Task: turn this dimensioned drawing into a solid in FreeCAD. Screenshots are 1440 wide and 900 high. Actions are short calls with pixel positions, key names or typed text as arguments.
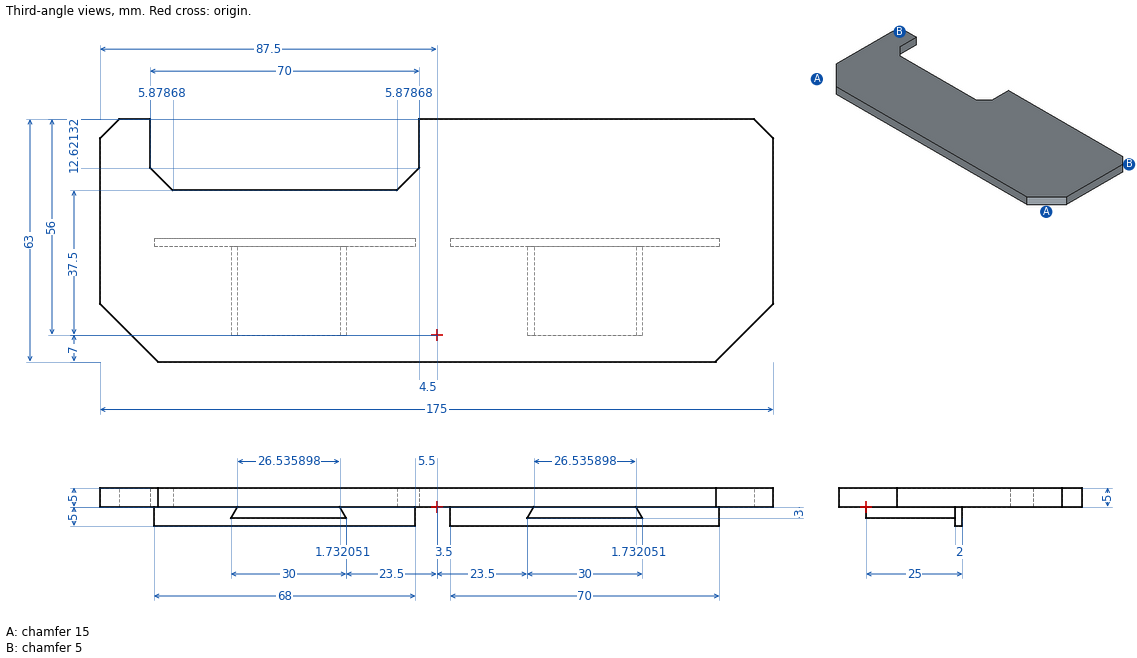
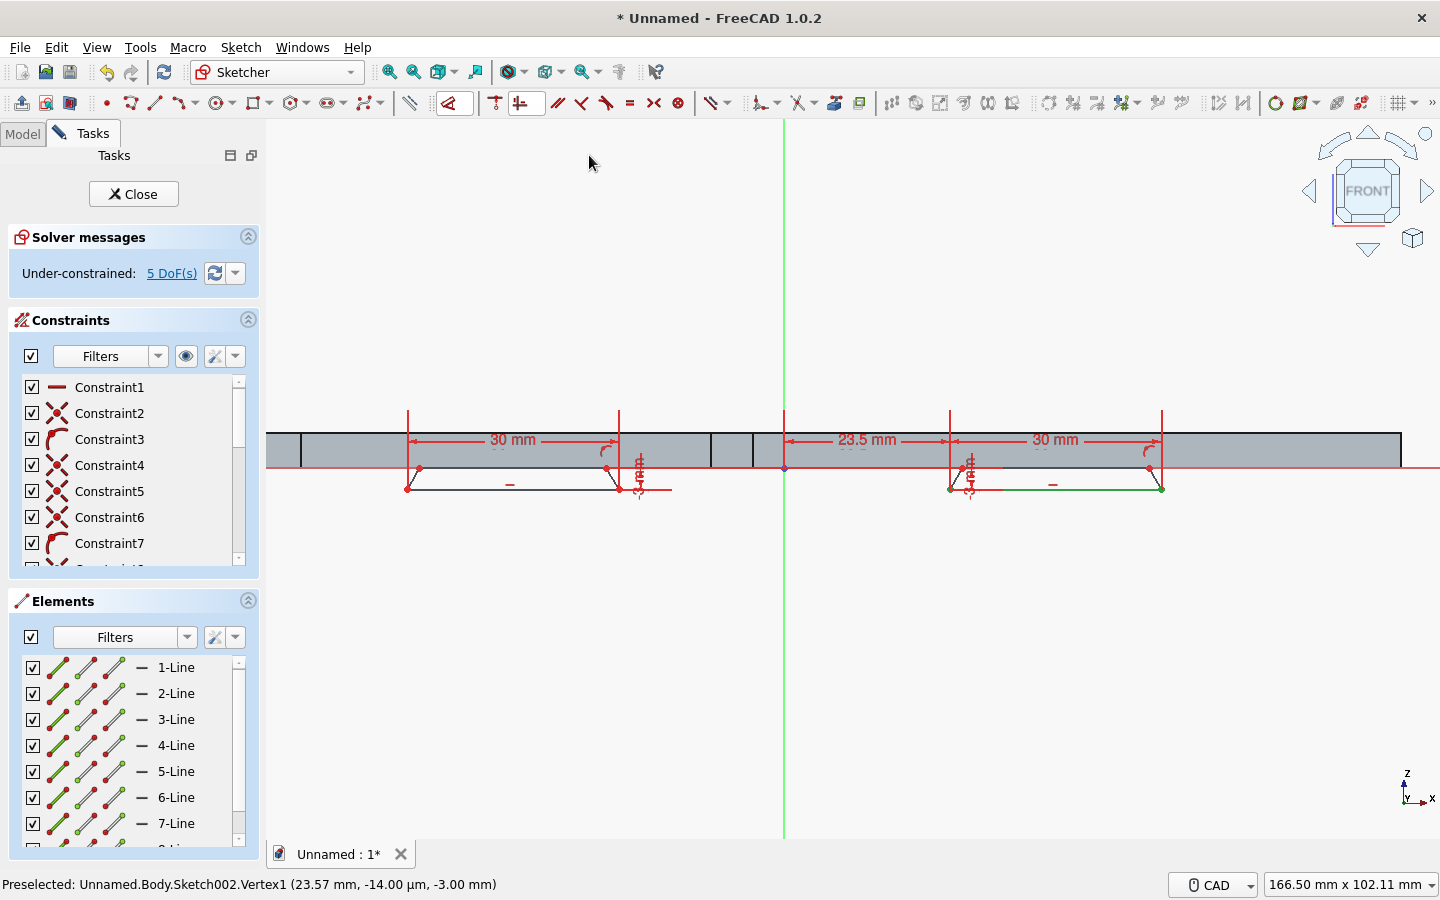
click(619, 490)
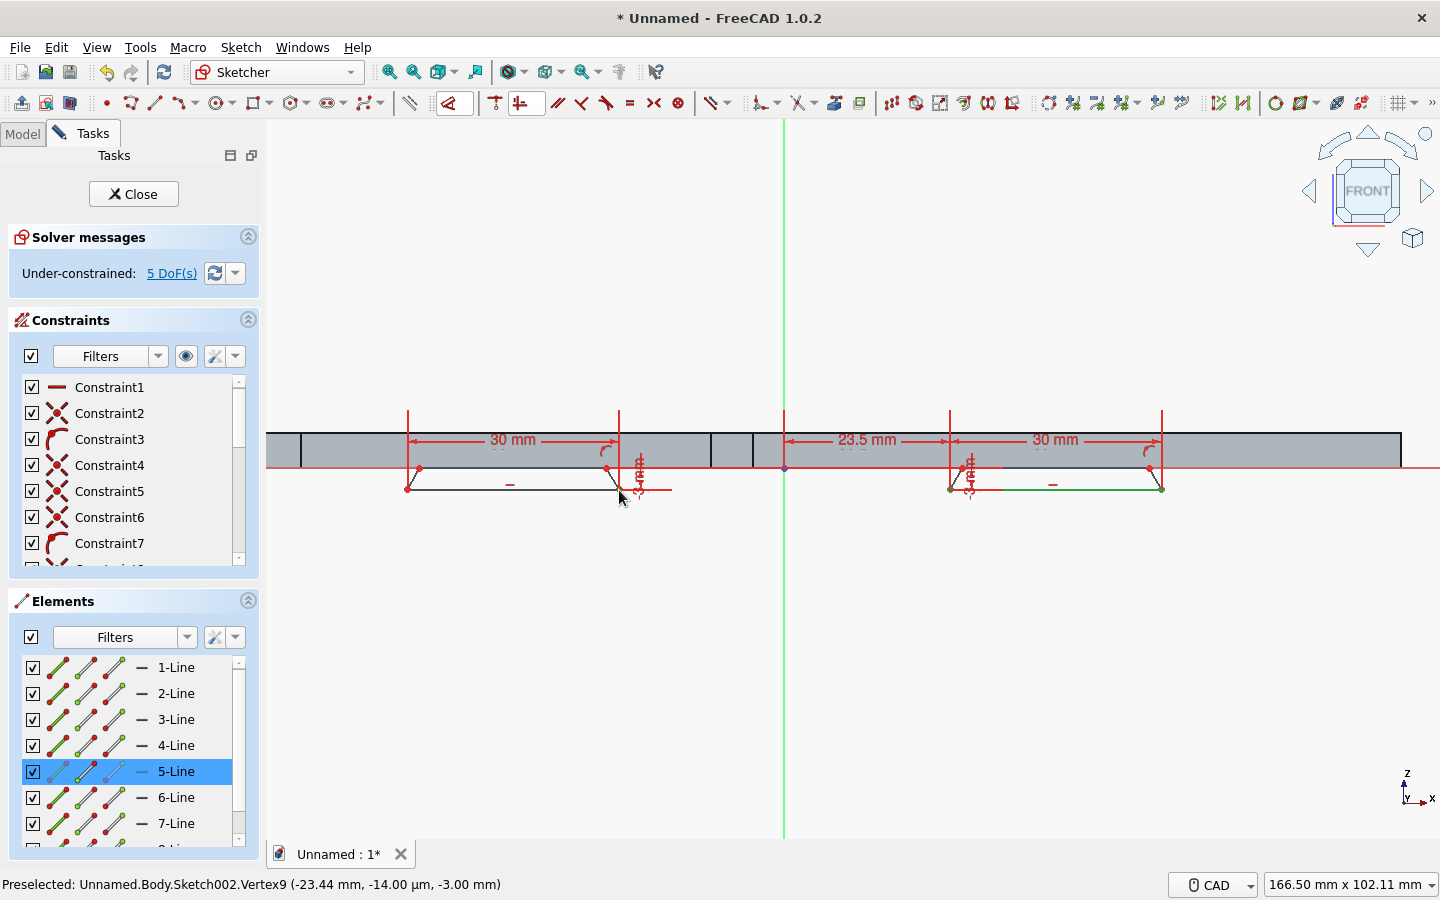
click(468, 104)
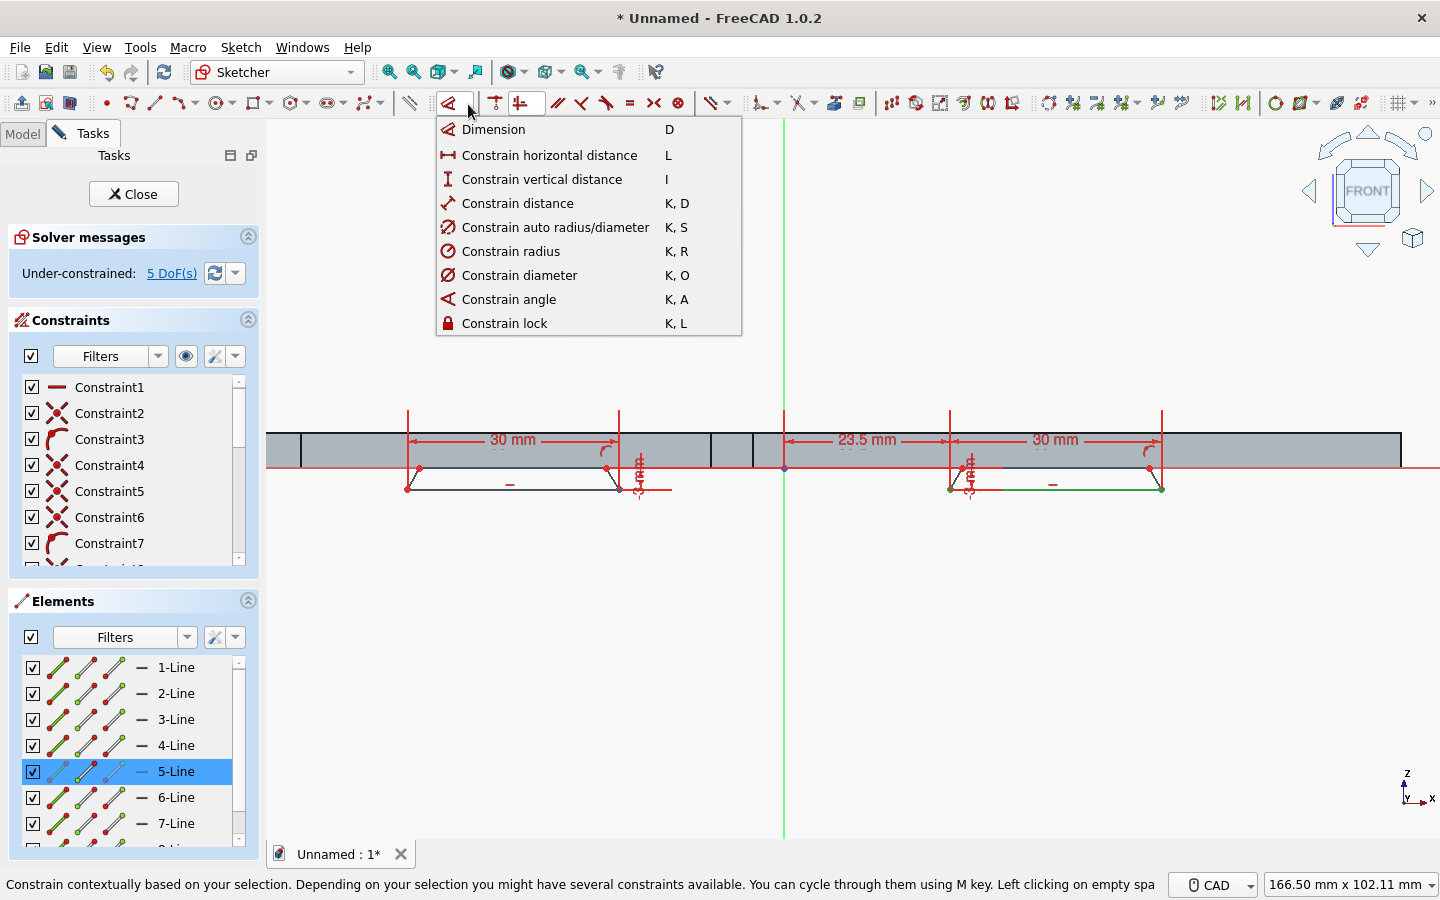
click(589, 155)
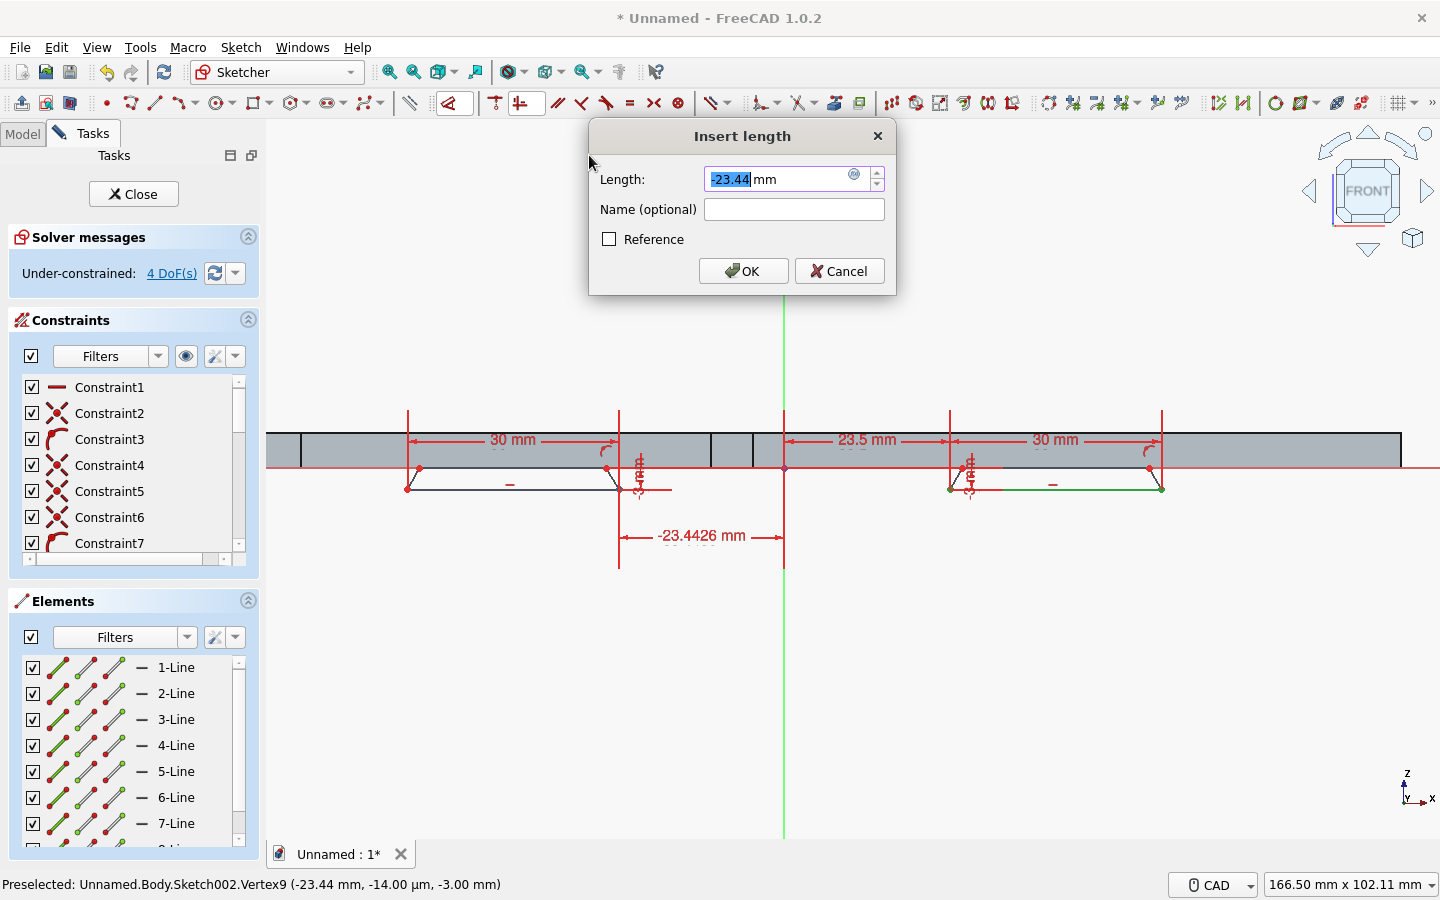
text(-23.5)
key(Return)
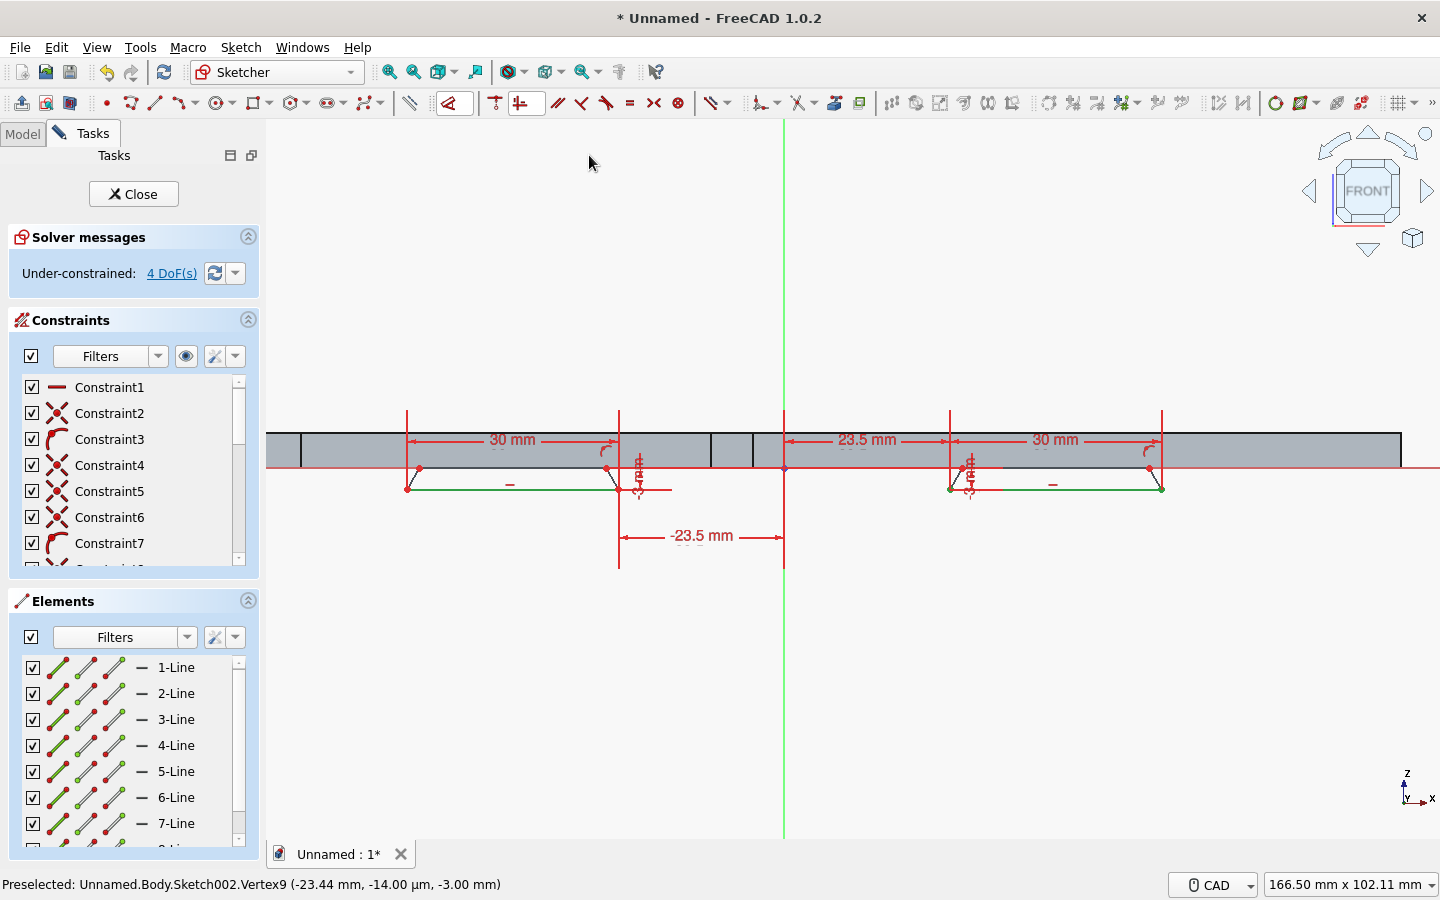
click(1093, 468)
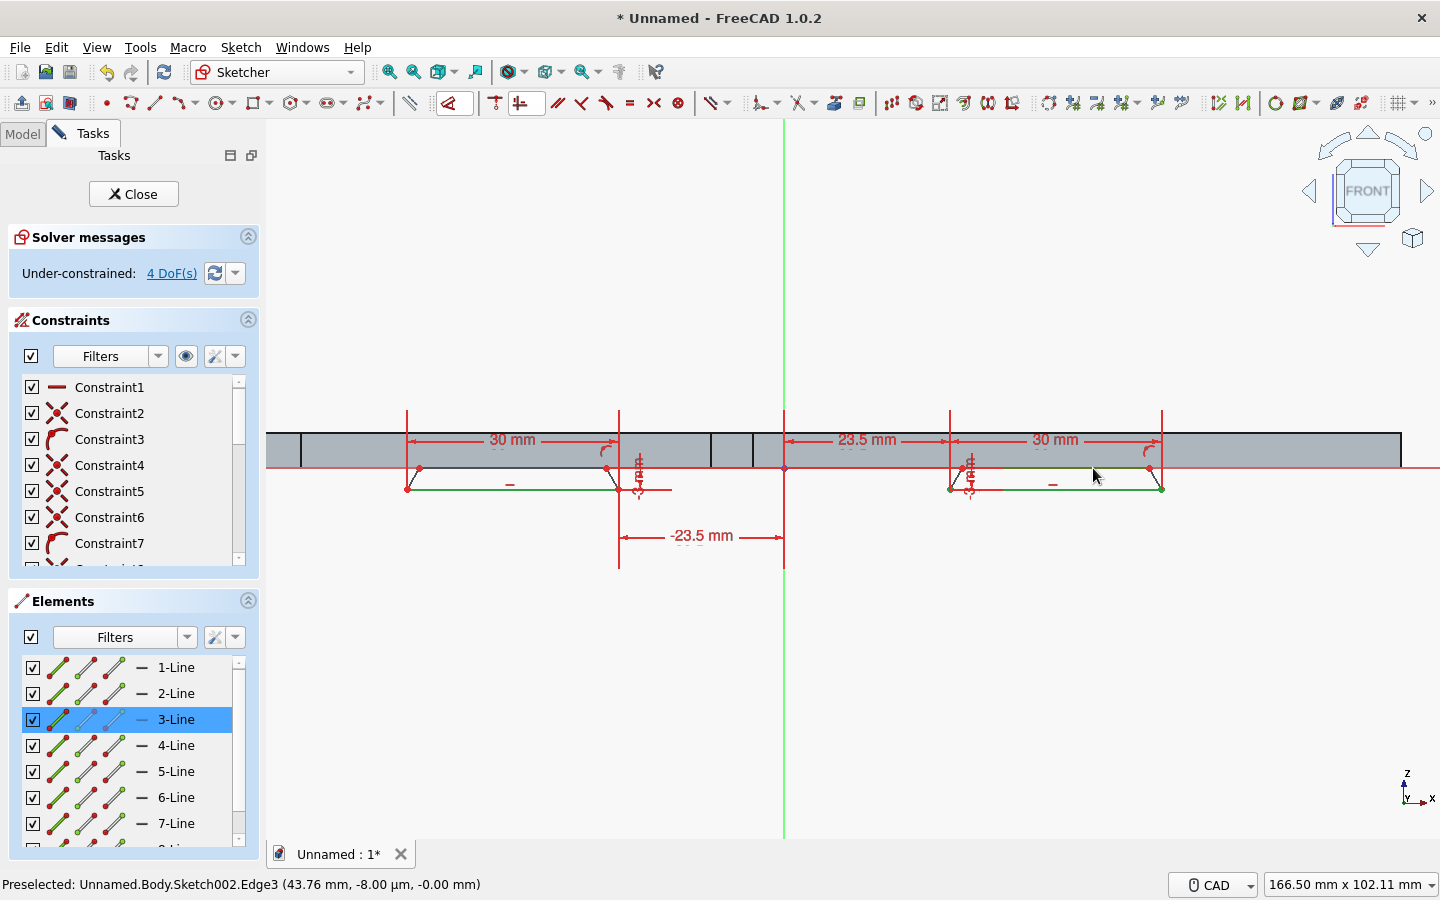
key(l)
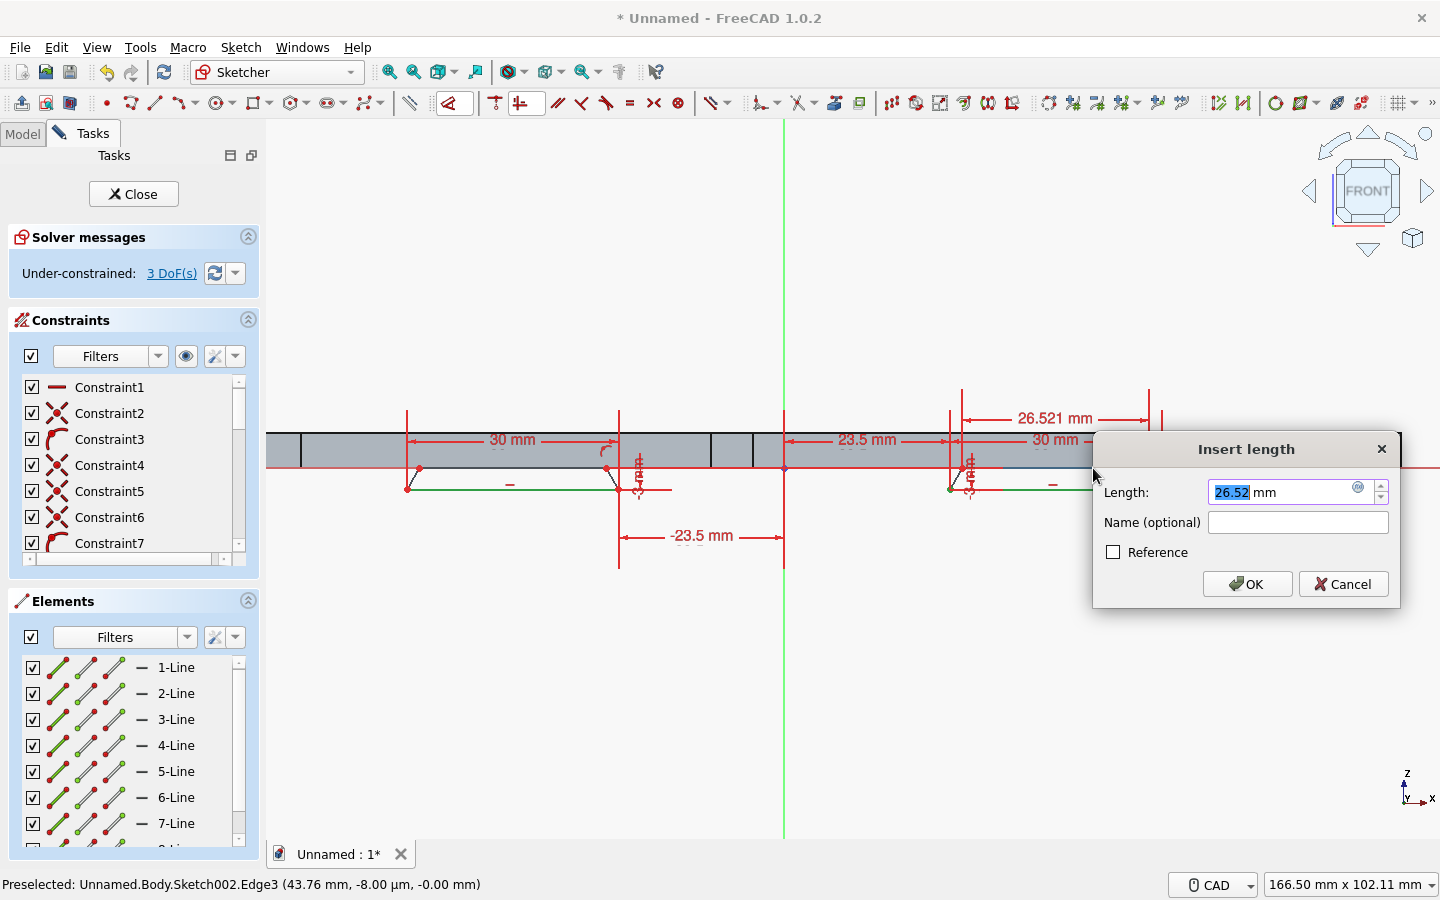
text(26.535898)
key(Return)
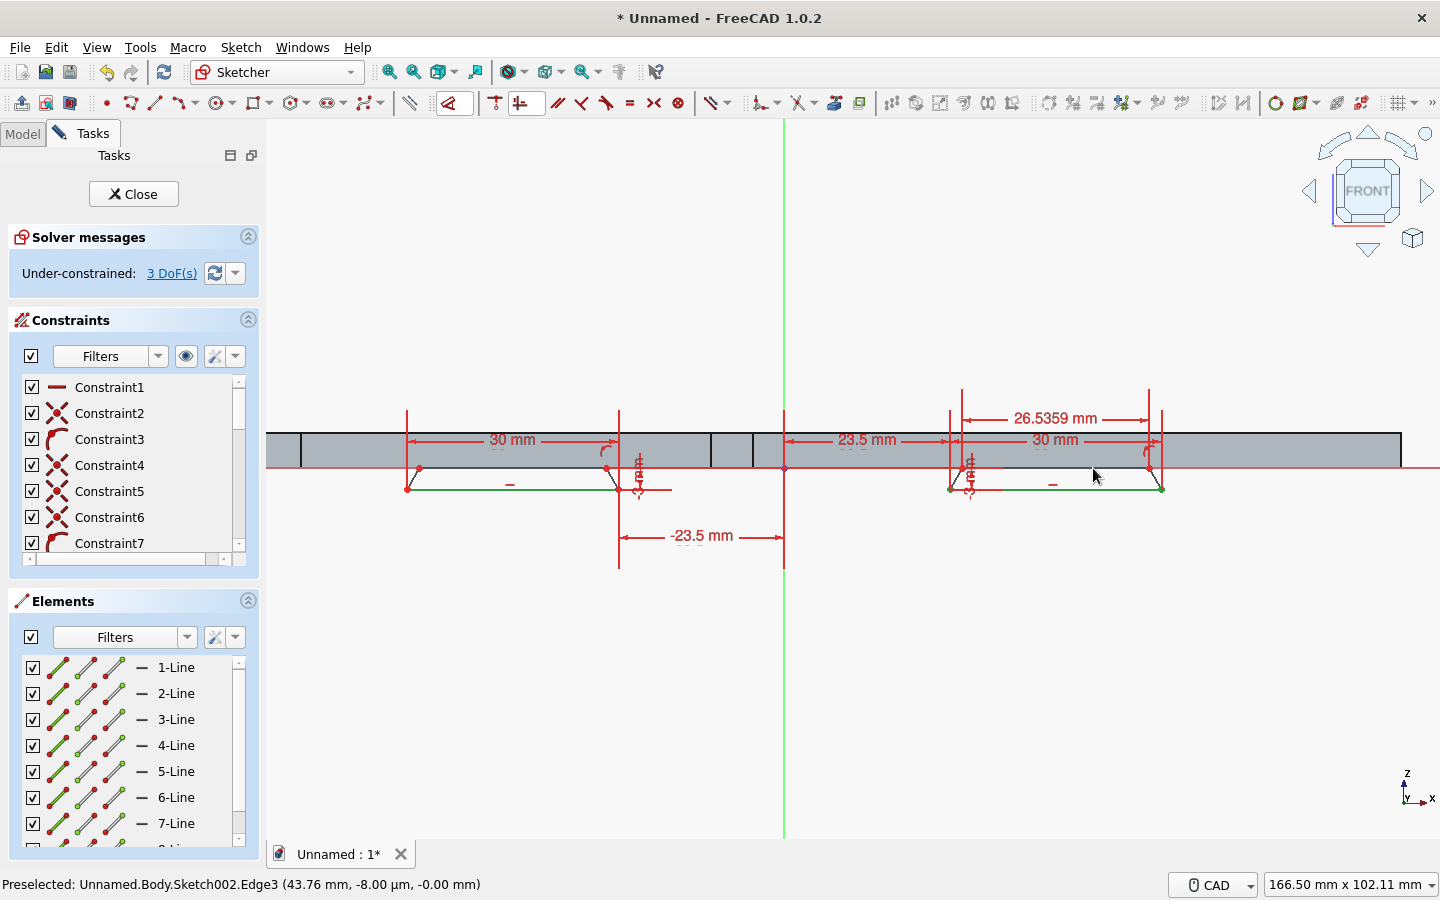
click(550, 468)